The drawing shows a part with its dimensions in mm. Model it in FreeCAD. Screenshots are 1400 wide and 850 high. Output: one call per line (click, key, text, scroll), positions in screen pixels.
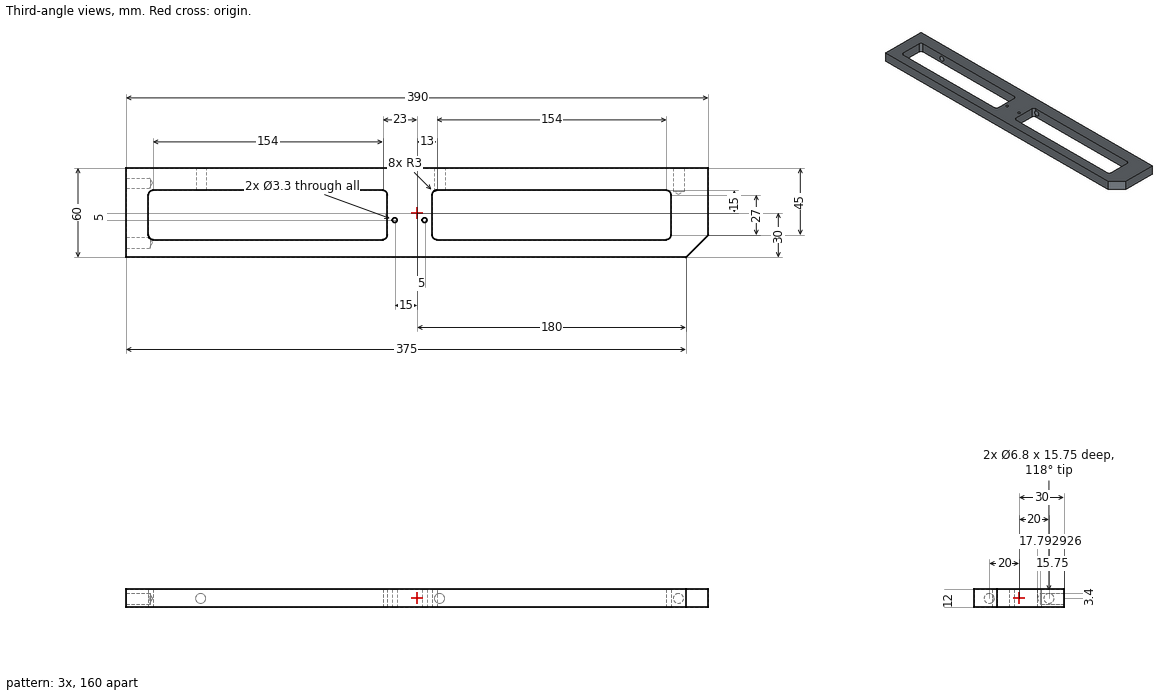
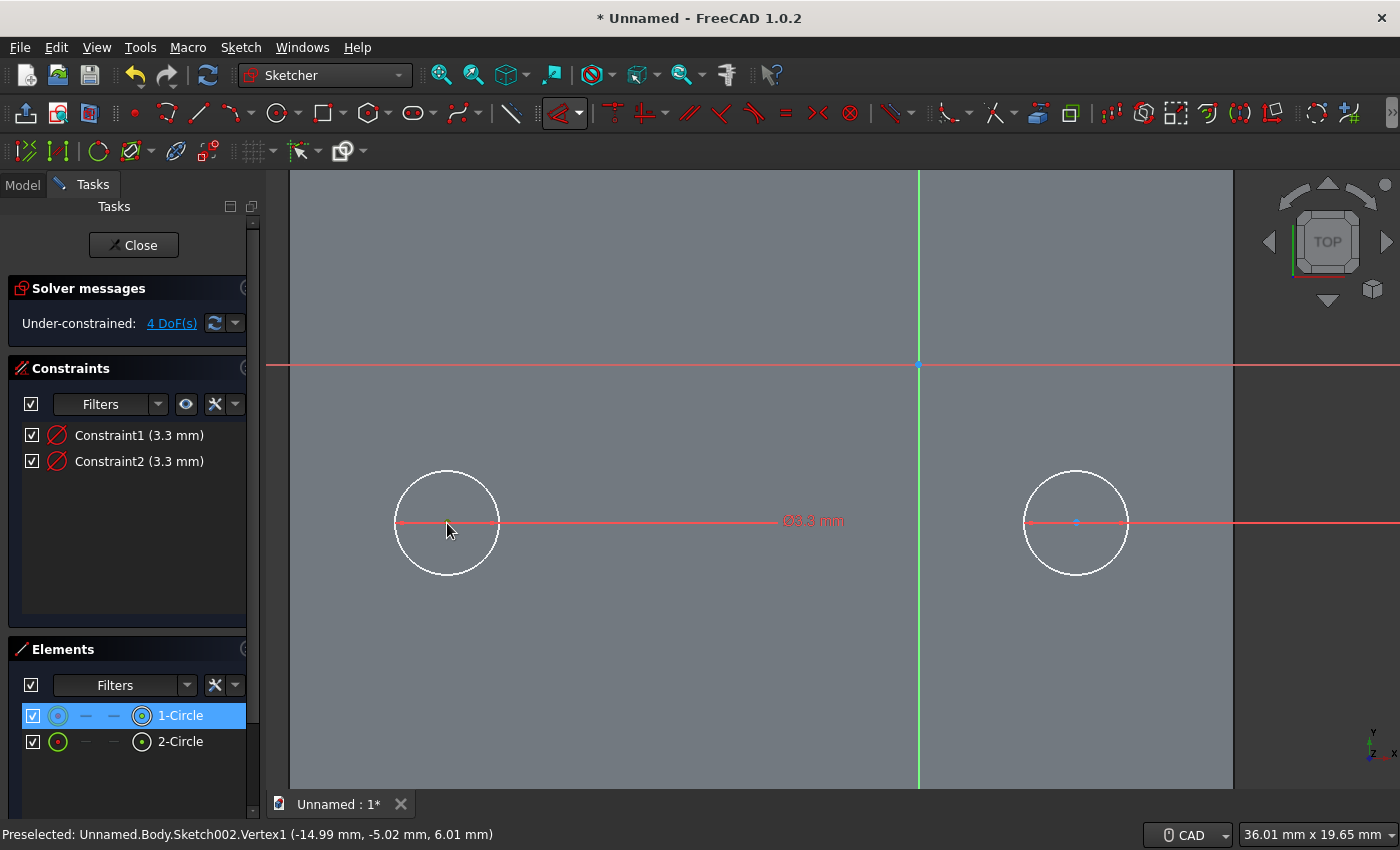
click(1076, 523)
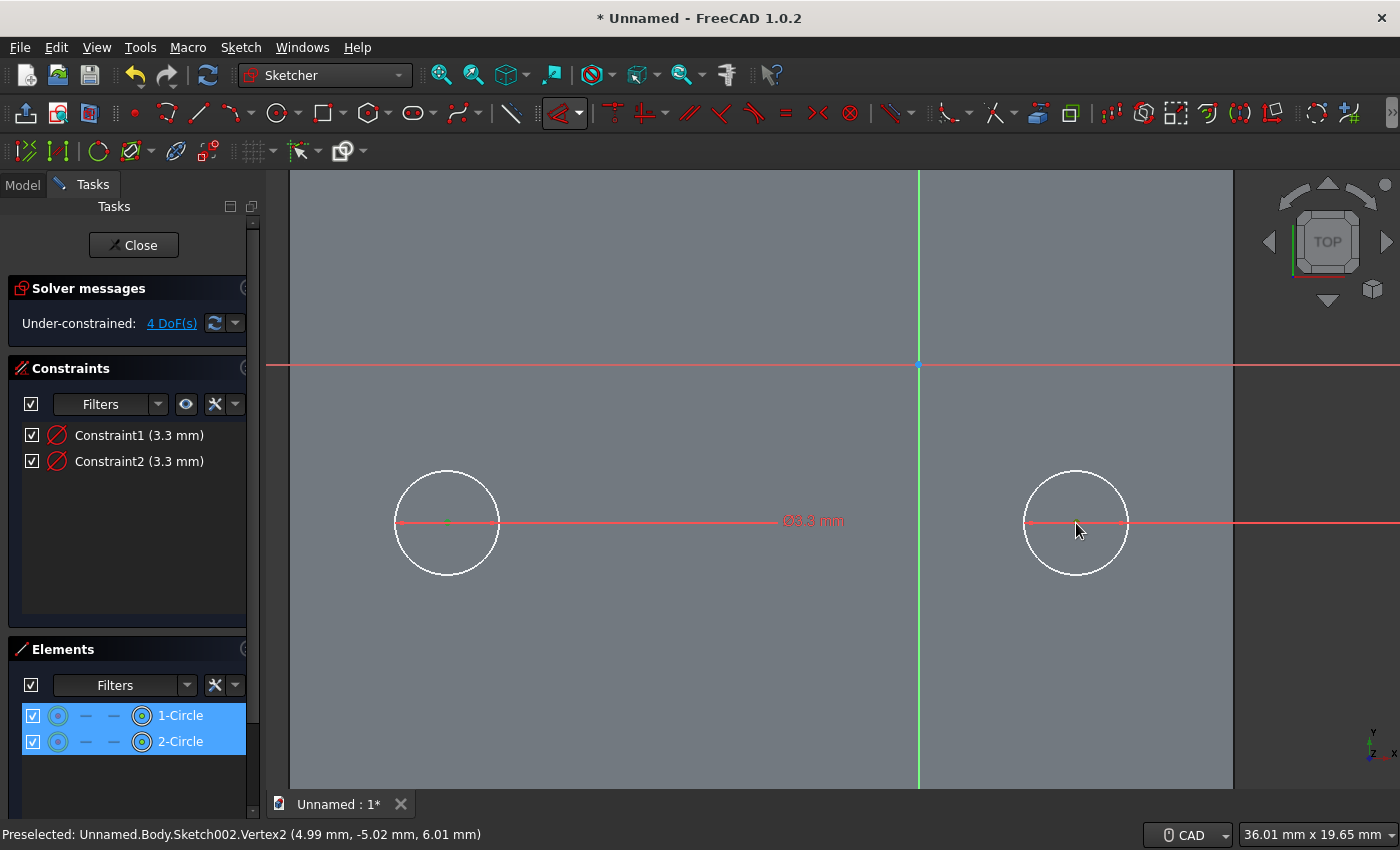
key(h)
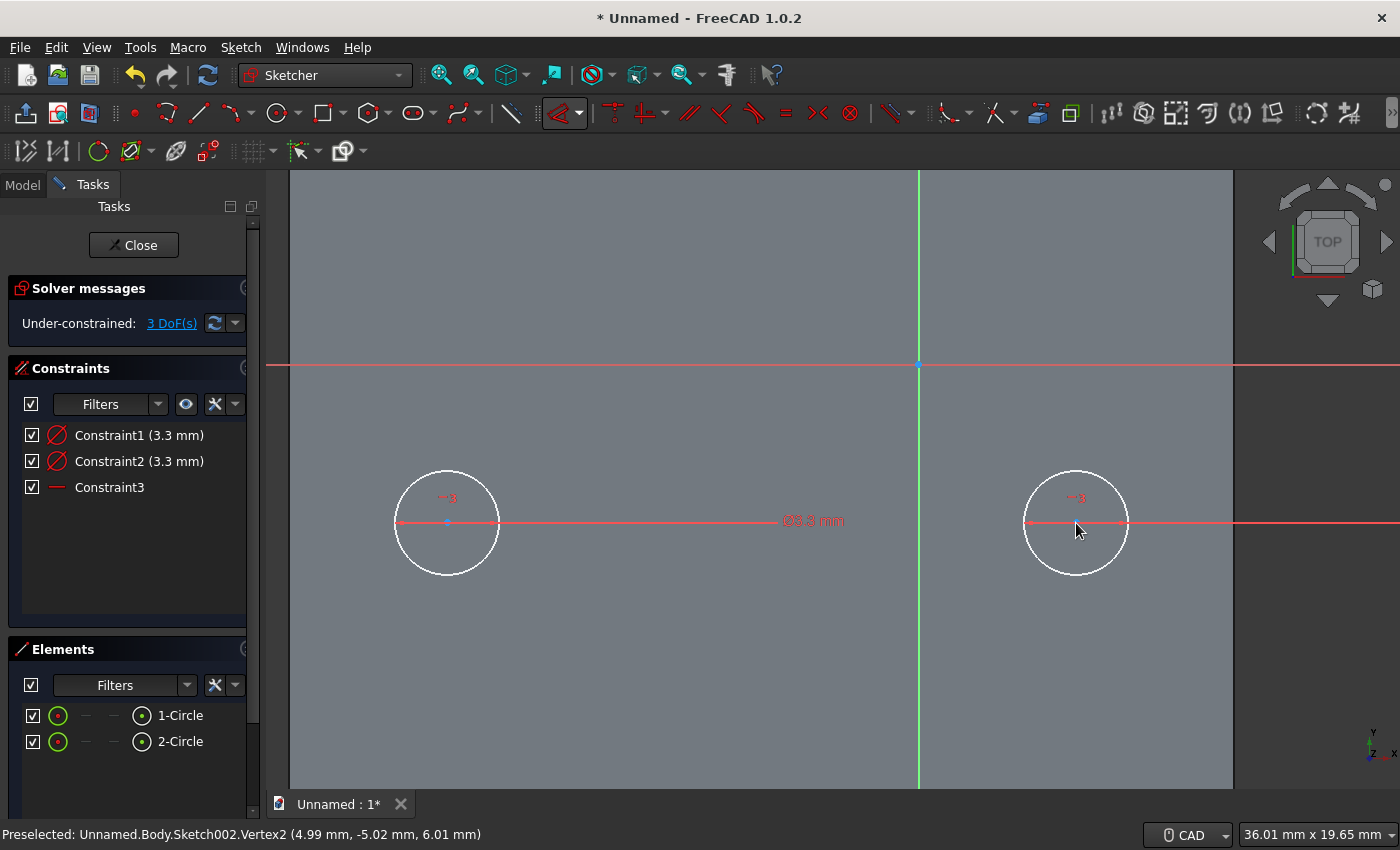
click(447, 523)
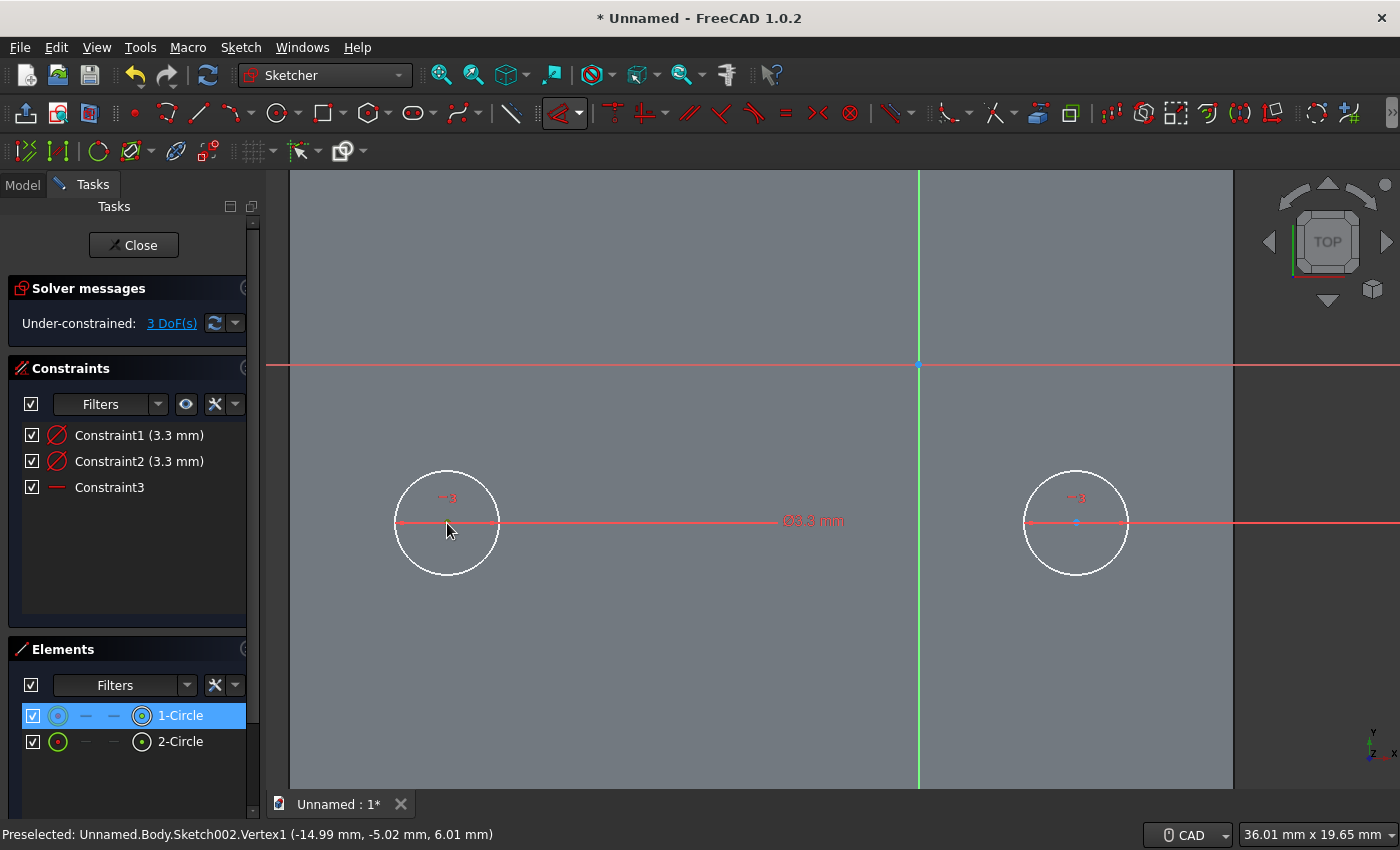
key(i)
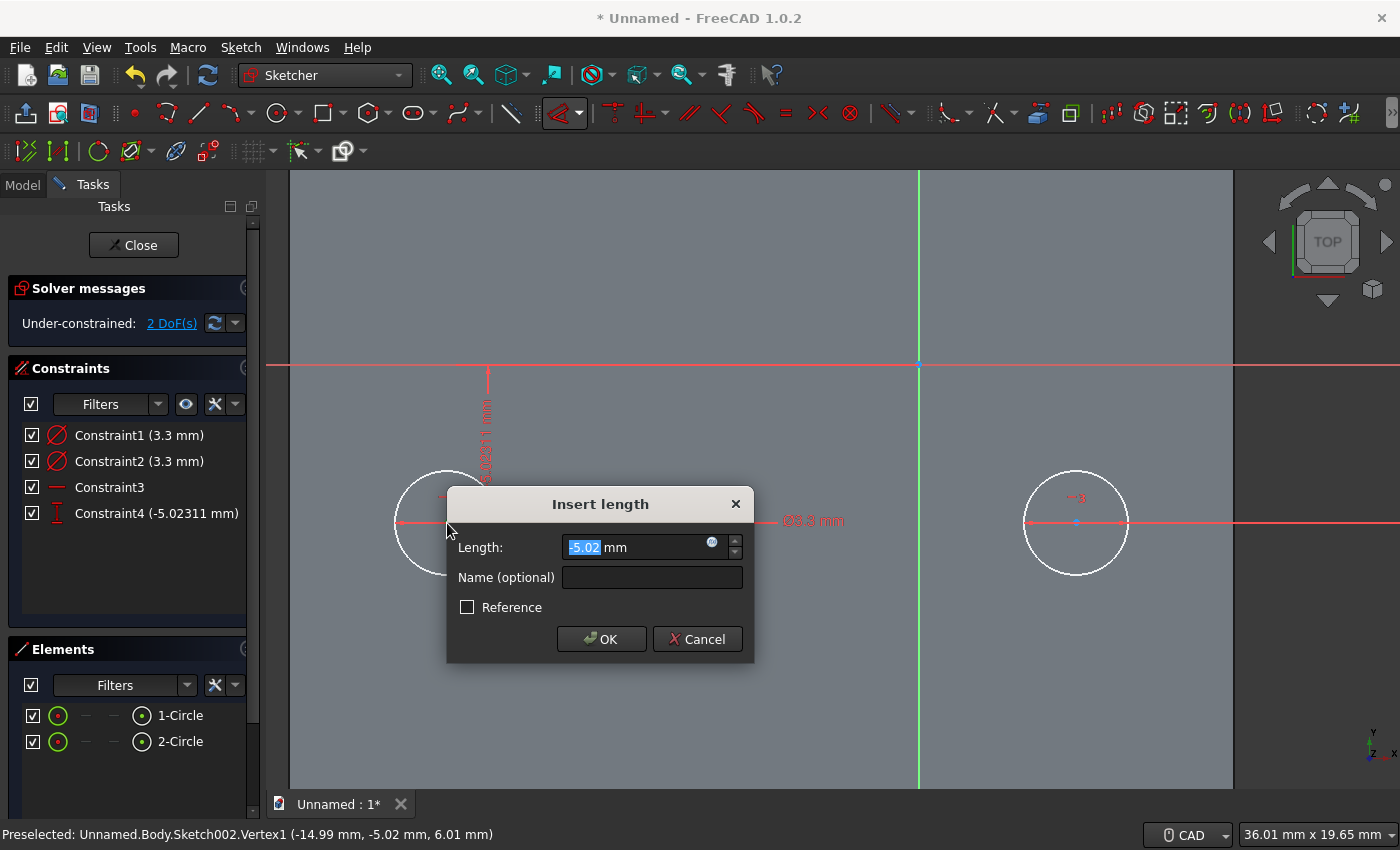
text(-5)
key(Return)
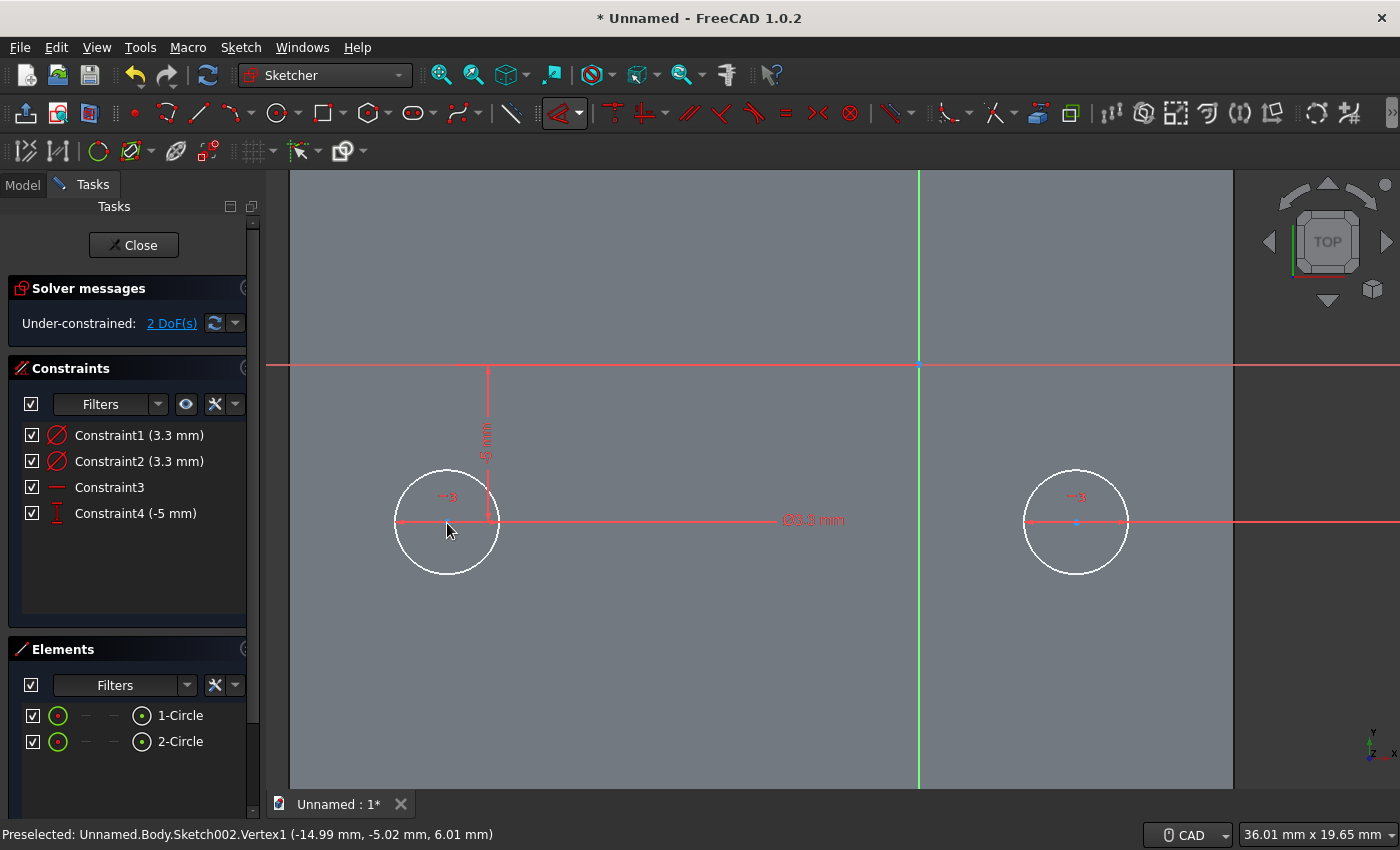
click(1076, 522)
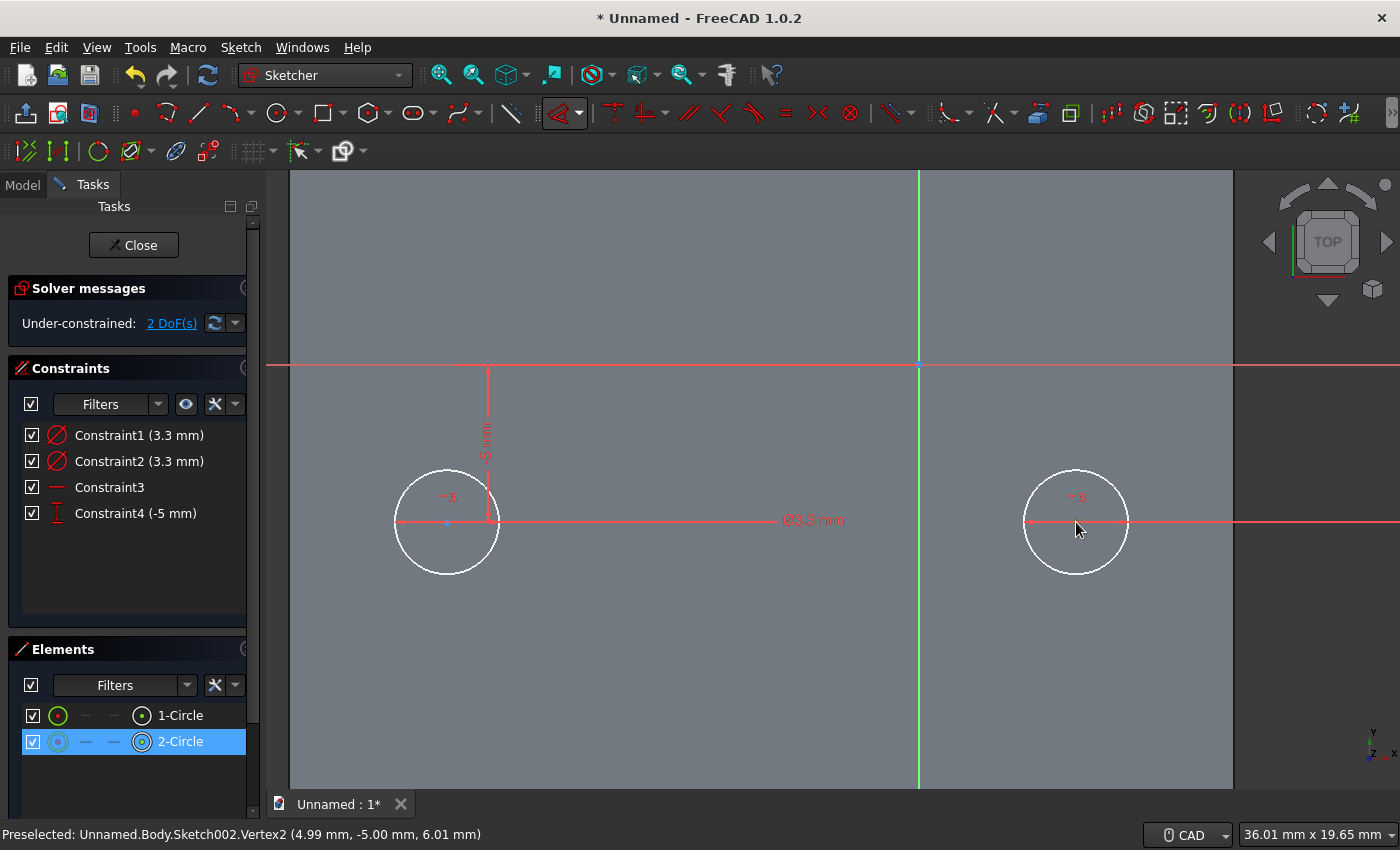
key(l)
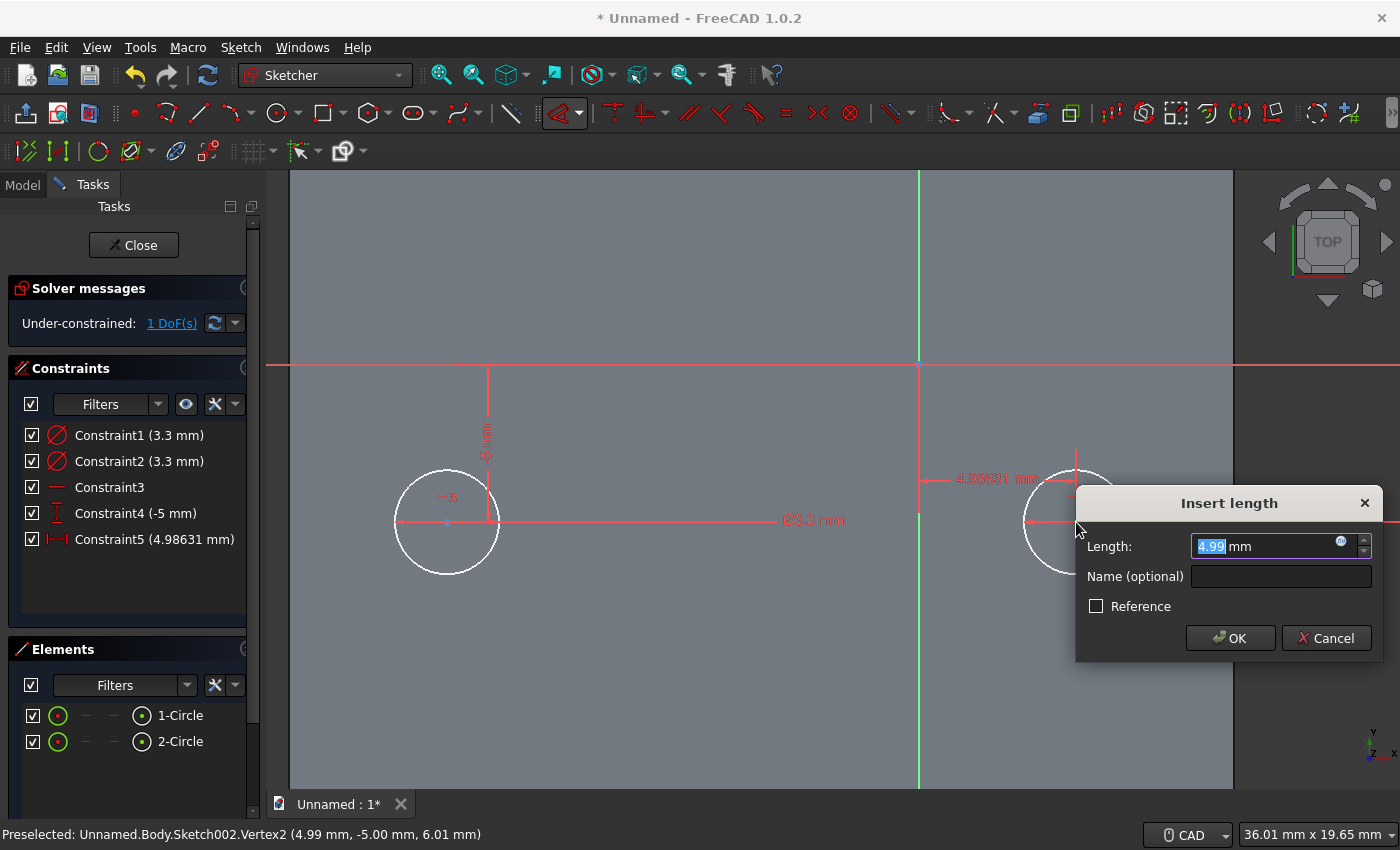
text(5)
key(Return)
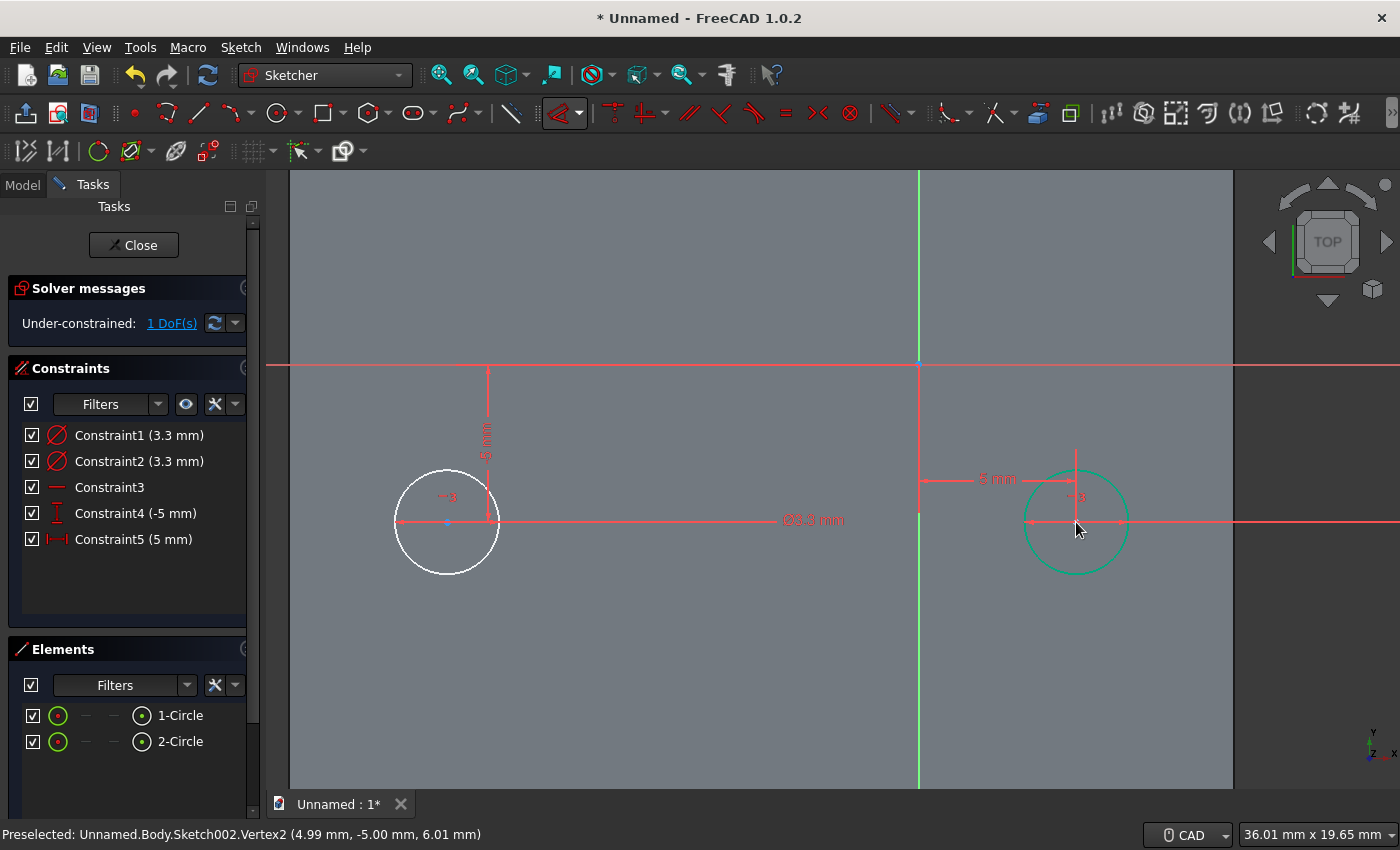
click(447, 522)